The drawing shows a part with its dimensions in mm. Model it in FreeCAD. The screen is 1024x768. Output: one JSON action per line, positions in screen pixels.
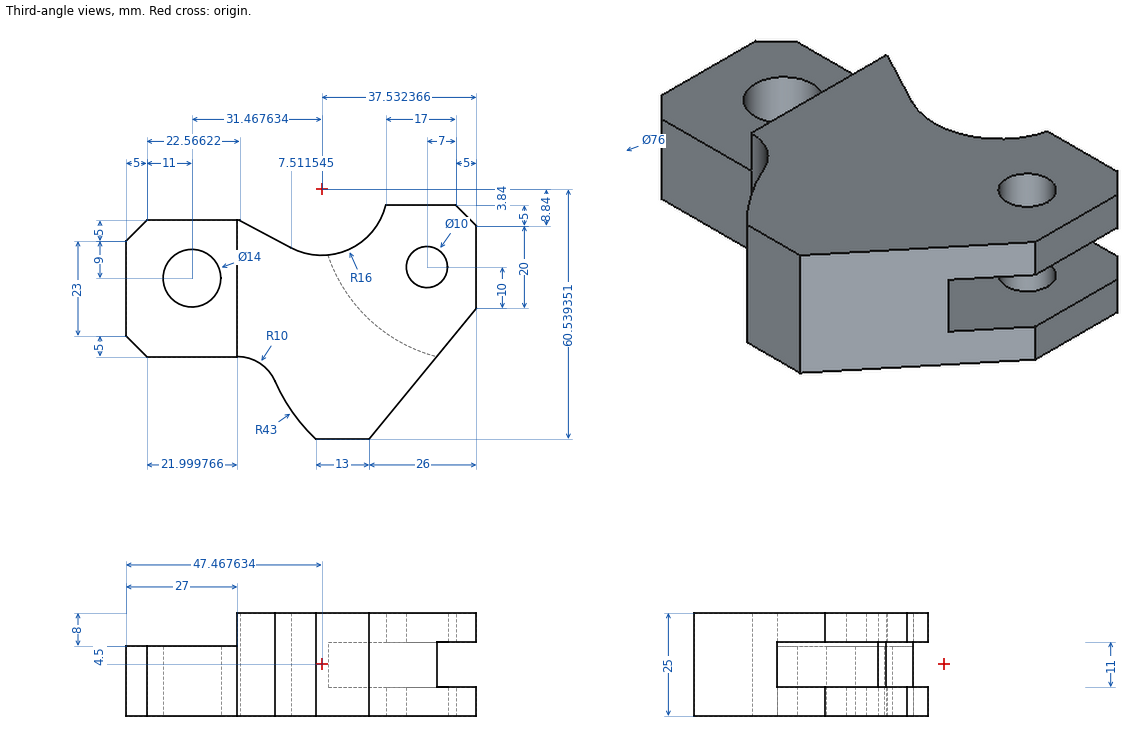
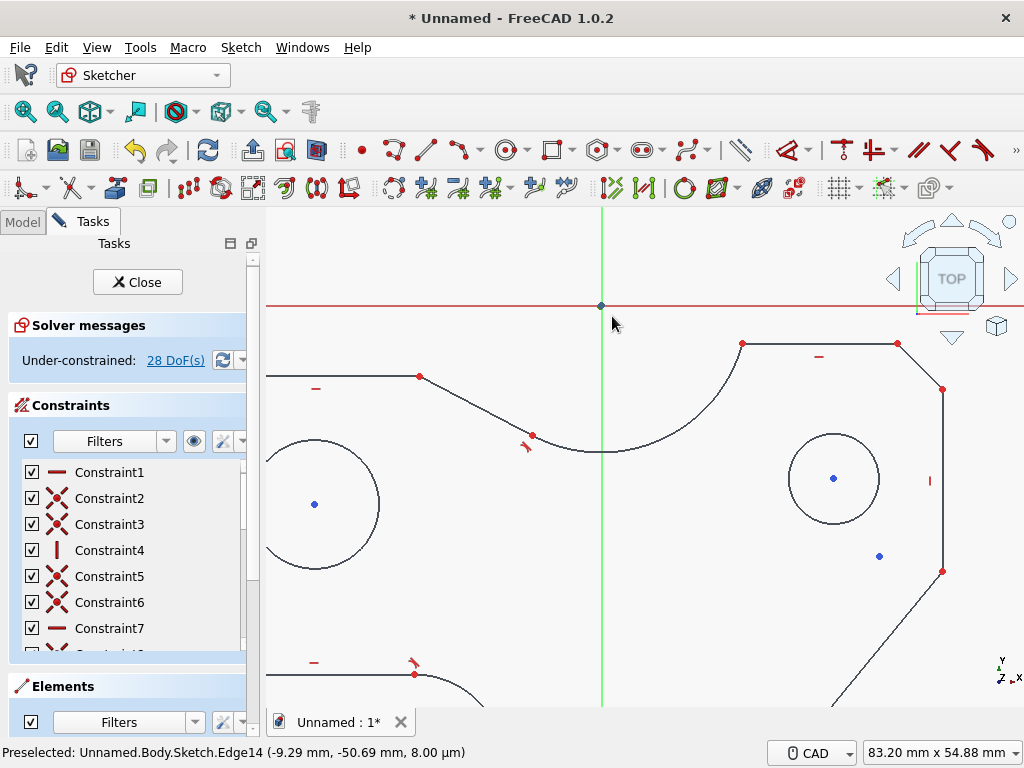
{"action": "left_click", "coordinate": [842, 150]}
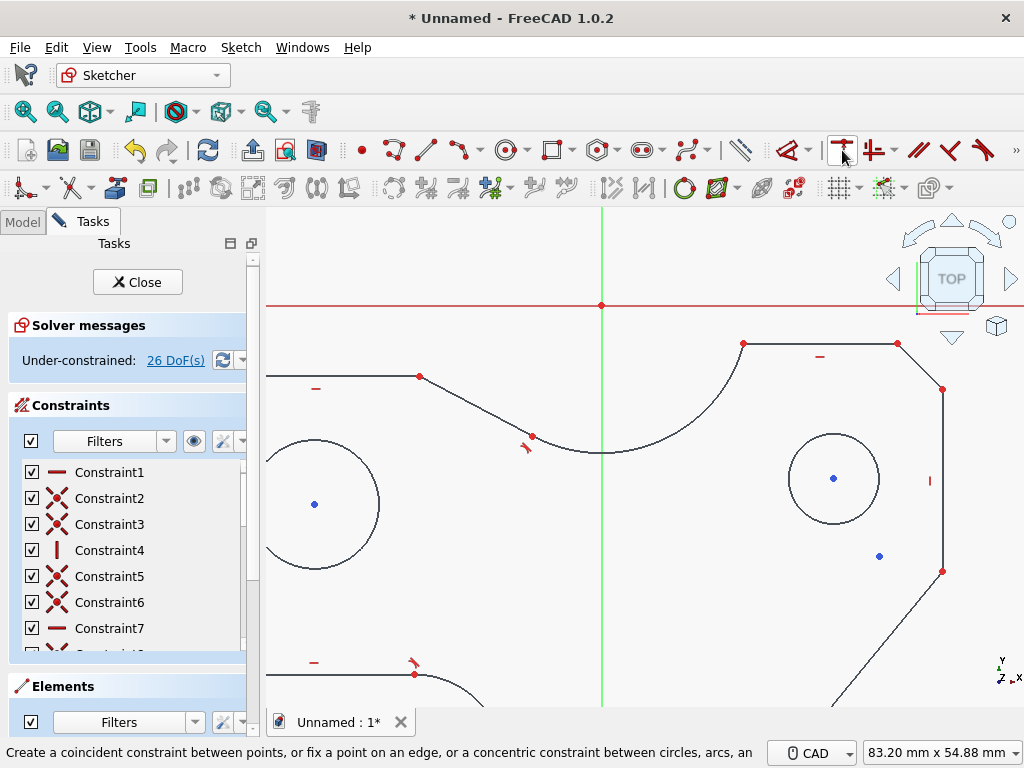
{"action": "left_click", "coordinate": [704, 411]}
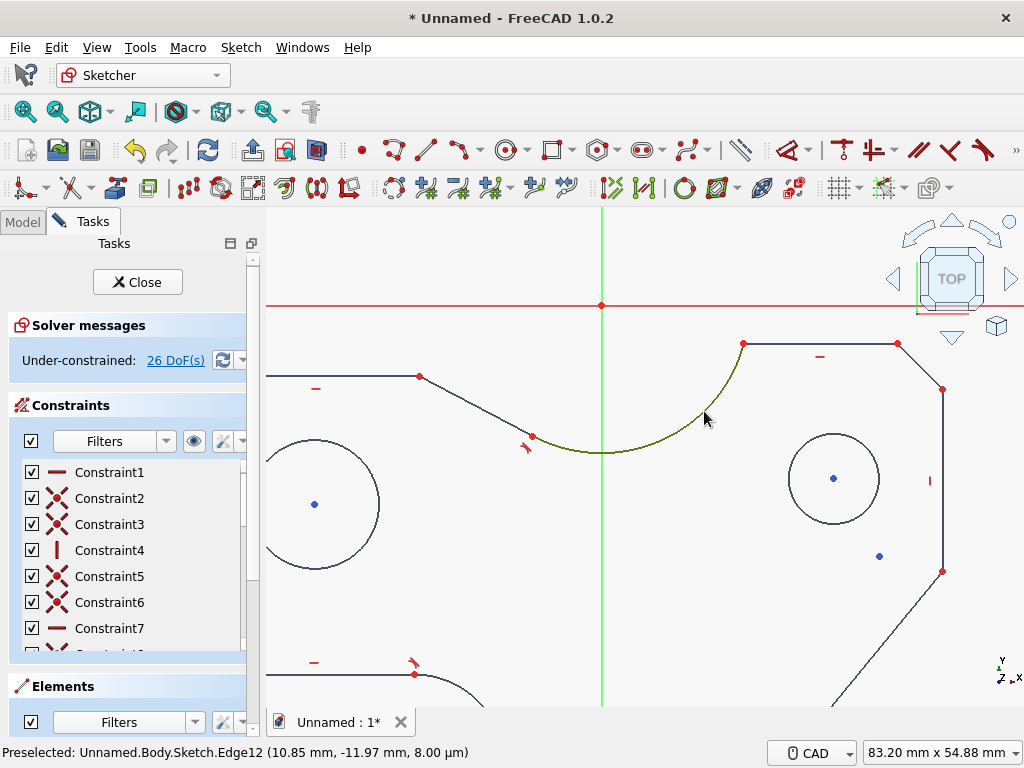
{"action": "key", "text": "k r"}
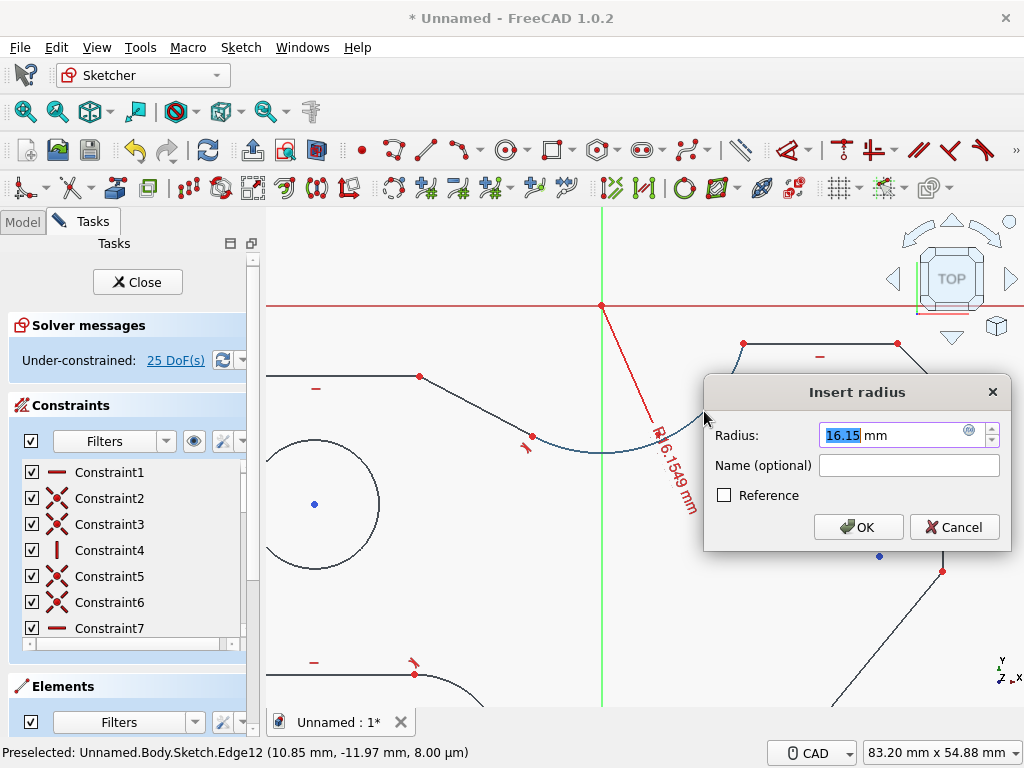
{"action": "type", "text": "16"}
{"action": "key", "text": "Return"}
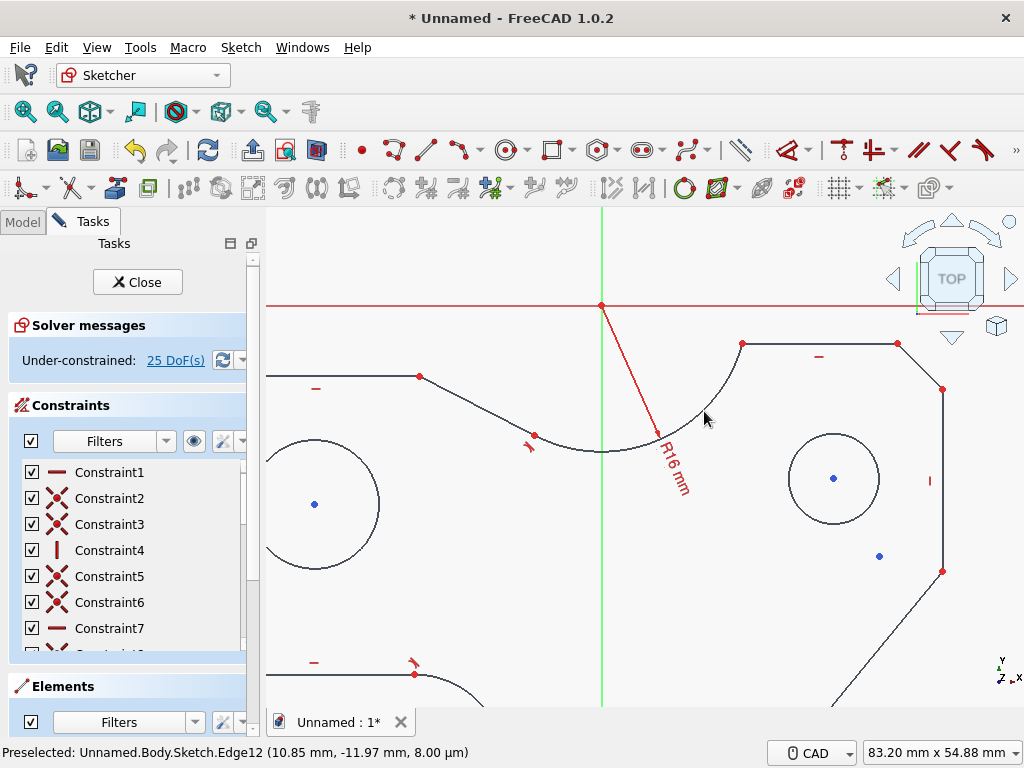
{"action": "left_click", "coordinate": [435, 677]}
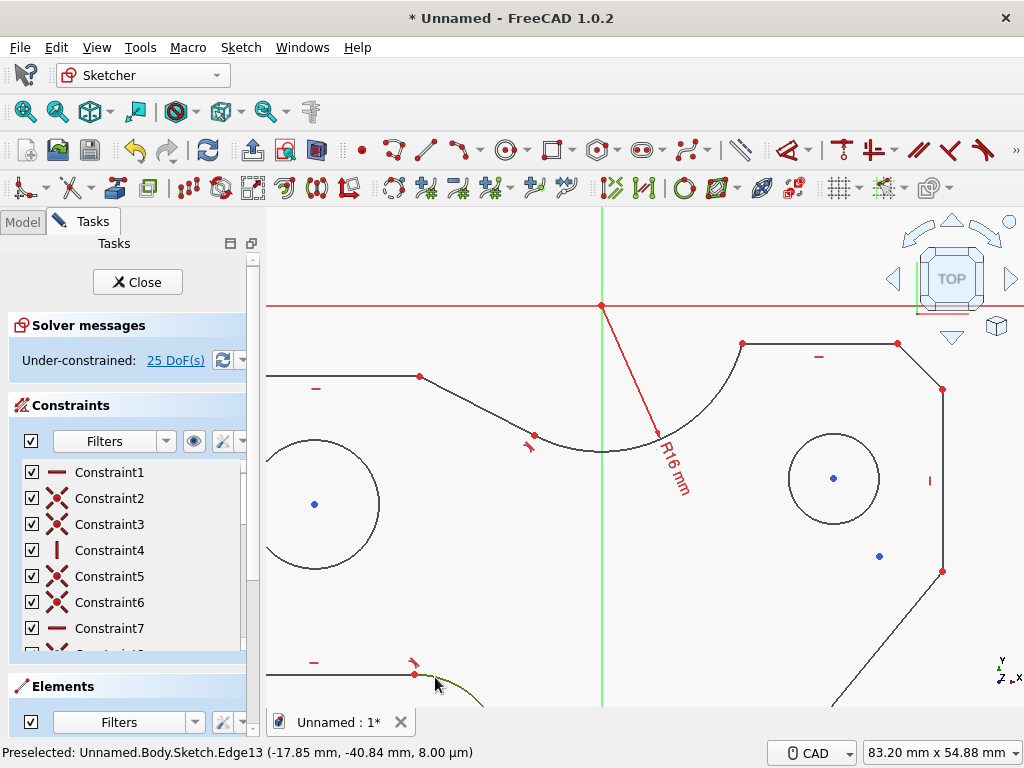
{"action": "left_click", "coordinate": [810, 150]}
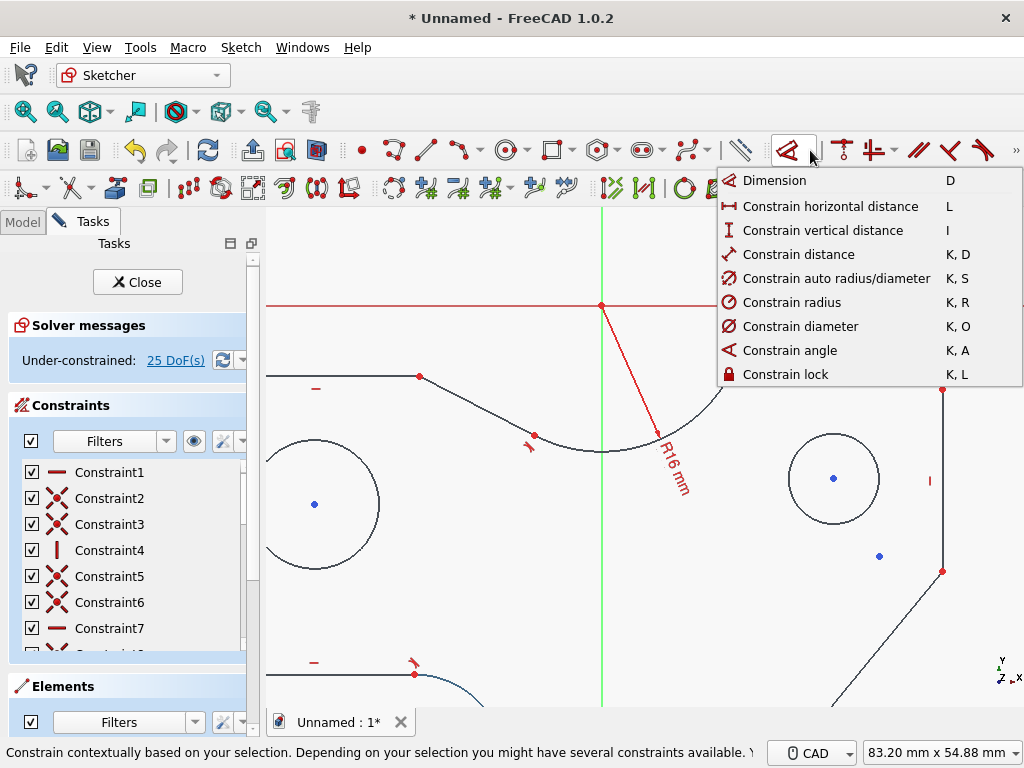
{"action": "left_click", "coordinate": [870, 302]}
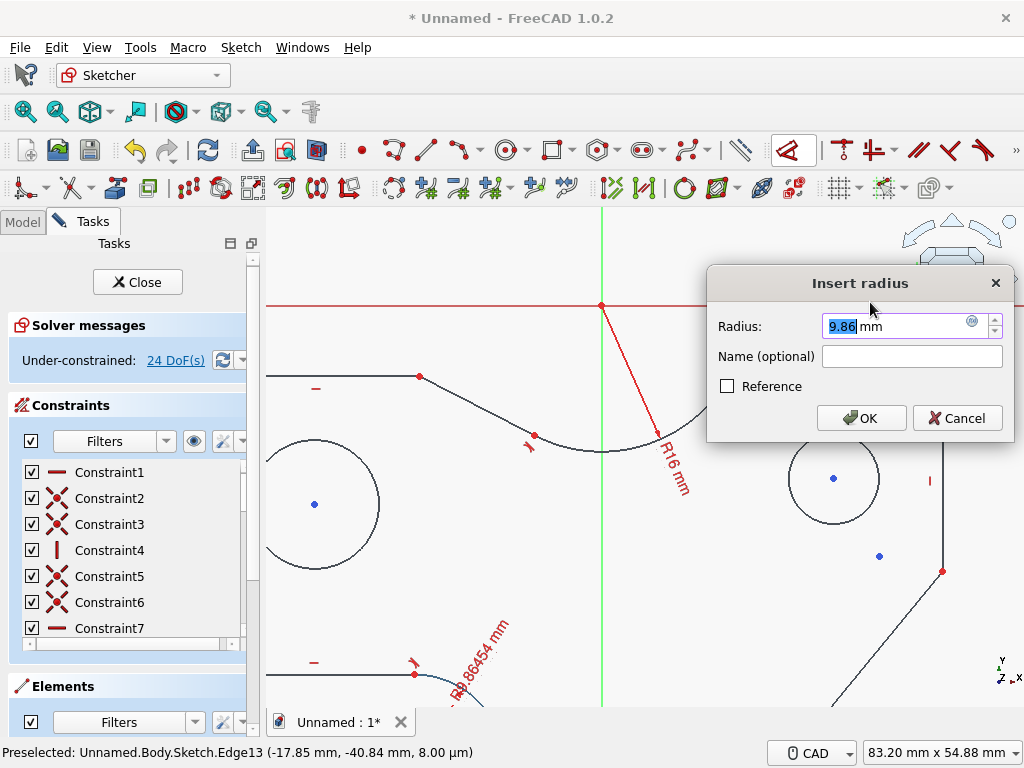
{"action": "type", "text": "10"}
{"action": "key", "text": "Return"}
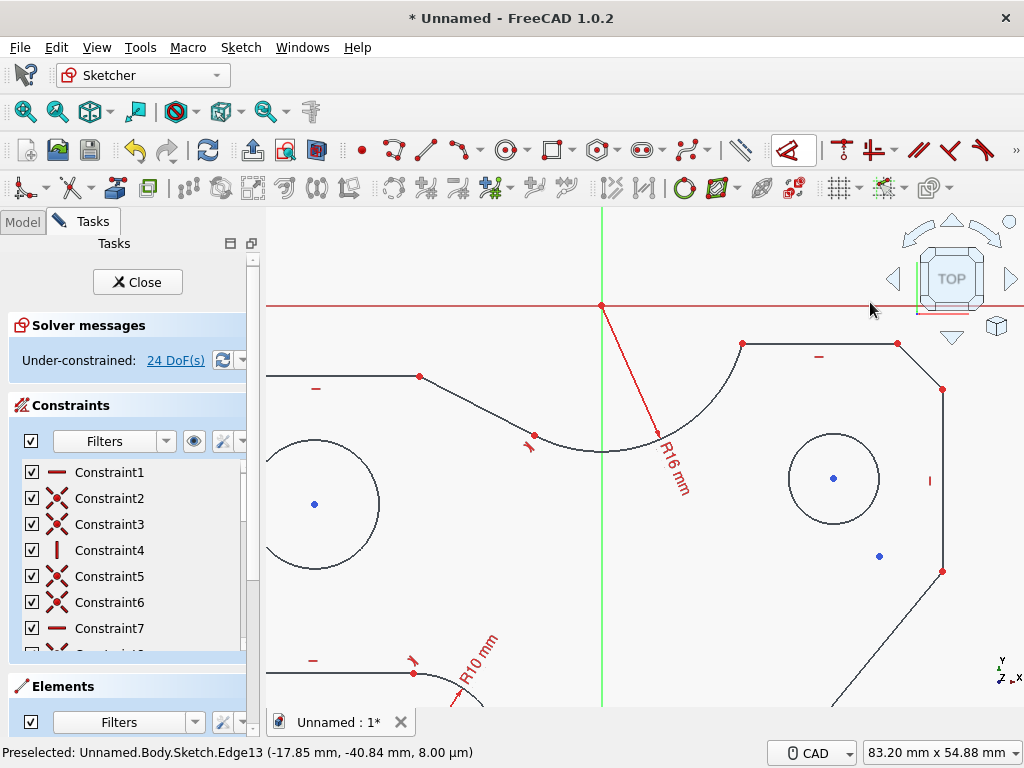
{"action": "scroll", "coordinate": [601, 305], "scroll_direction": "down", "scroll_amount": 3}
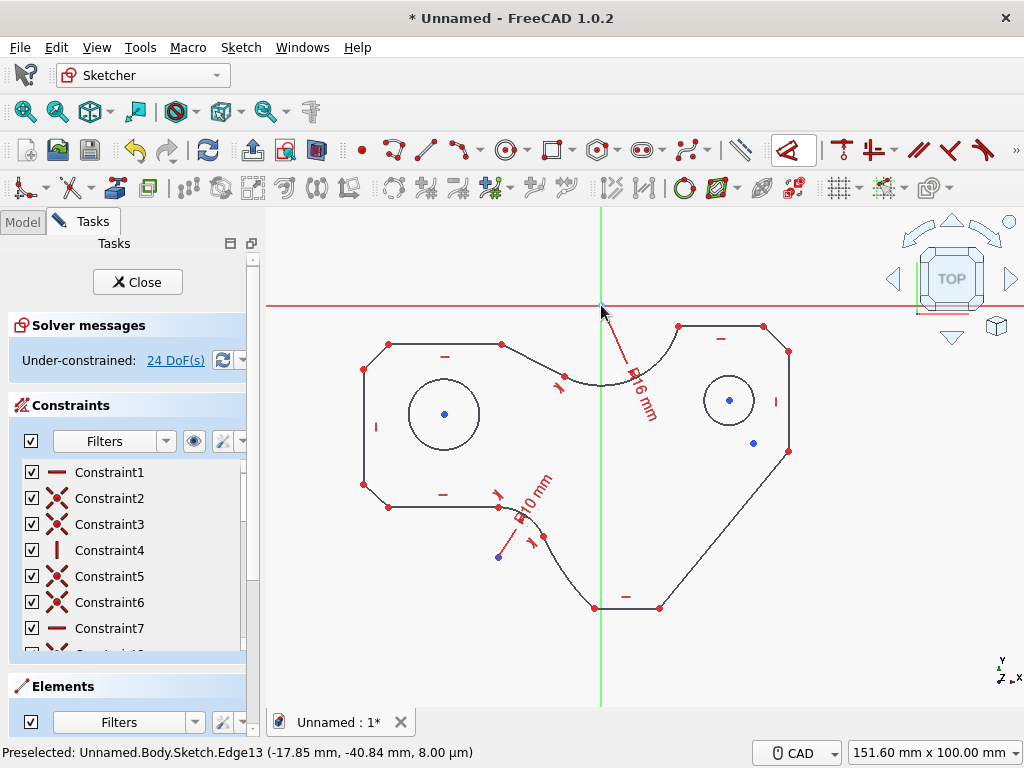
{"action": "left_click", "coordinate": [556, 560]}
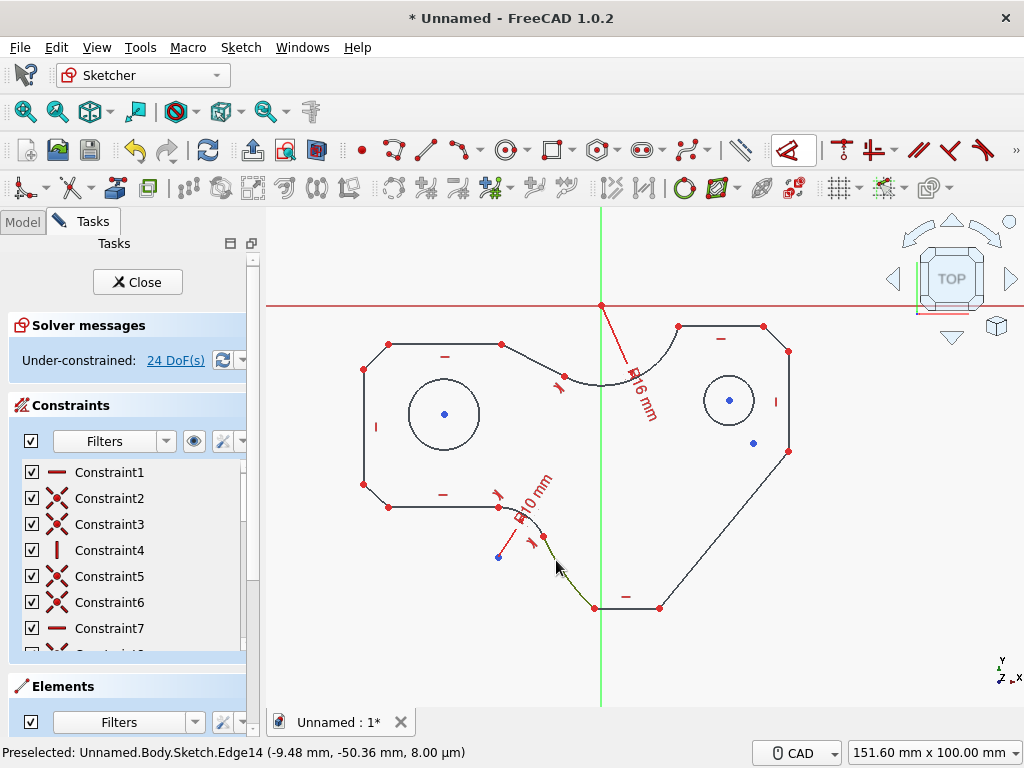
{"action": "left_click", "coordinate": [810, 150]}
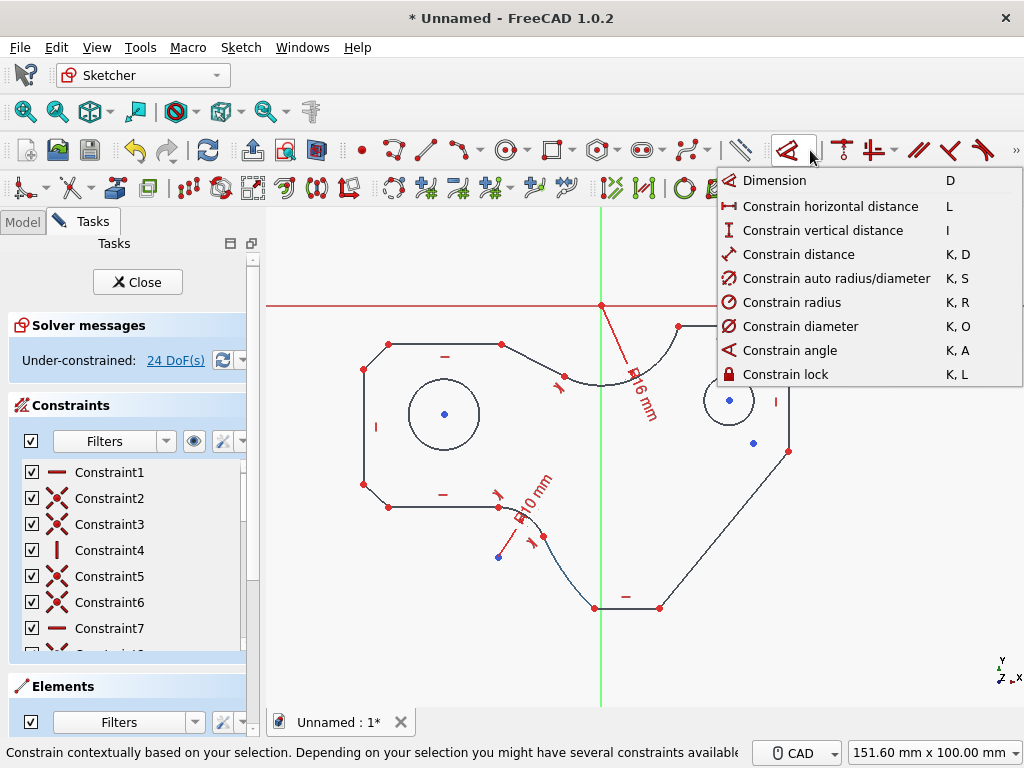
{"action": "left_click", "coordinate": [870, 302]}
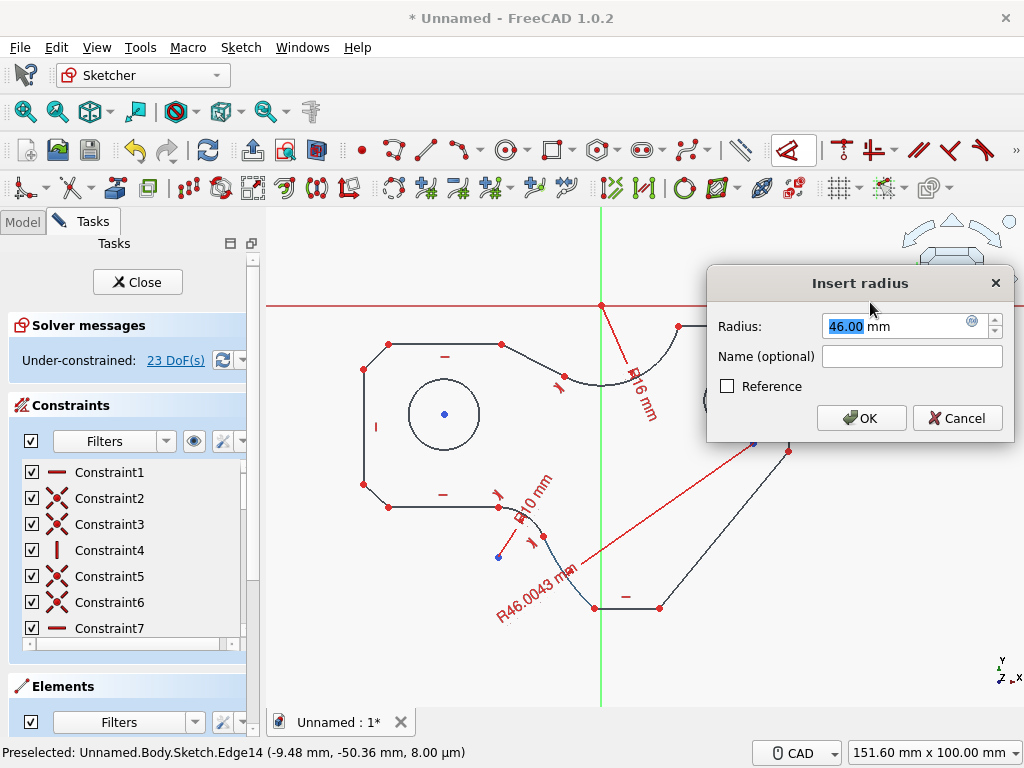
{"action": "type", "text": "43"}
{"action": "key", "text": "Return"}